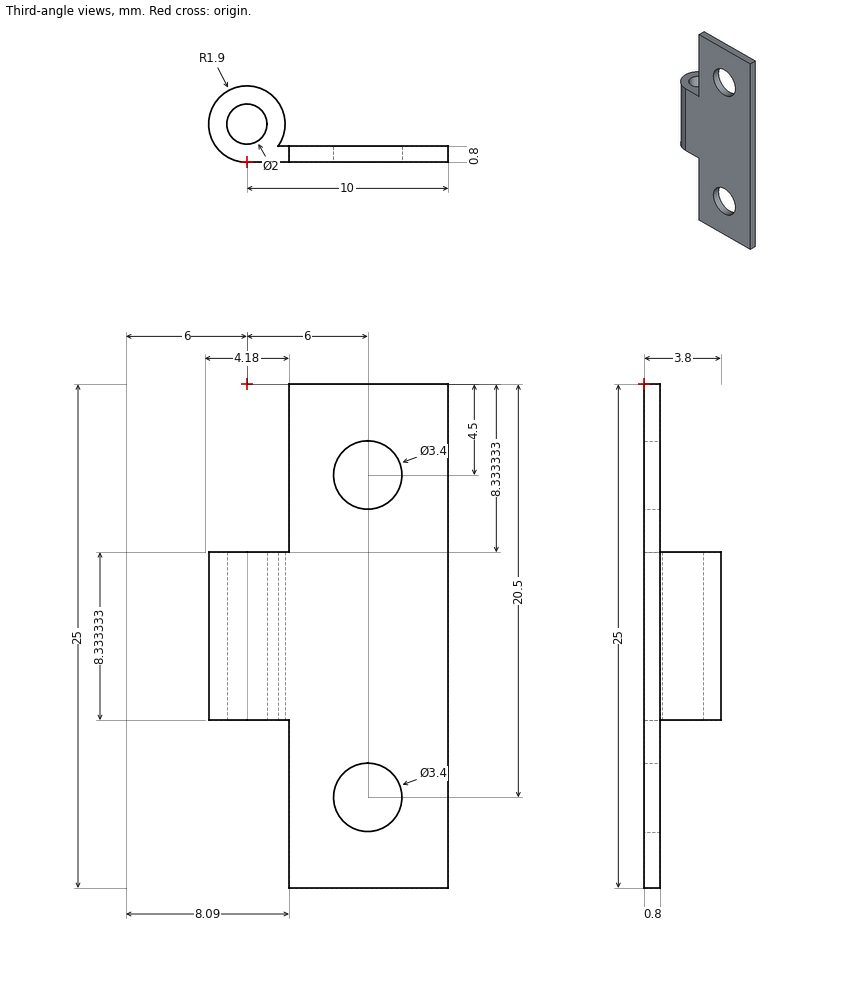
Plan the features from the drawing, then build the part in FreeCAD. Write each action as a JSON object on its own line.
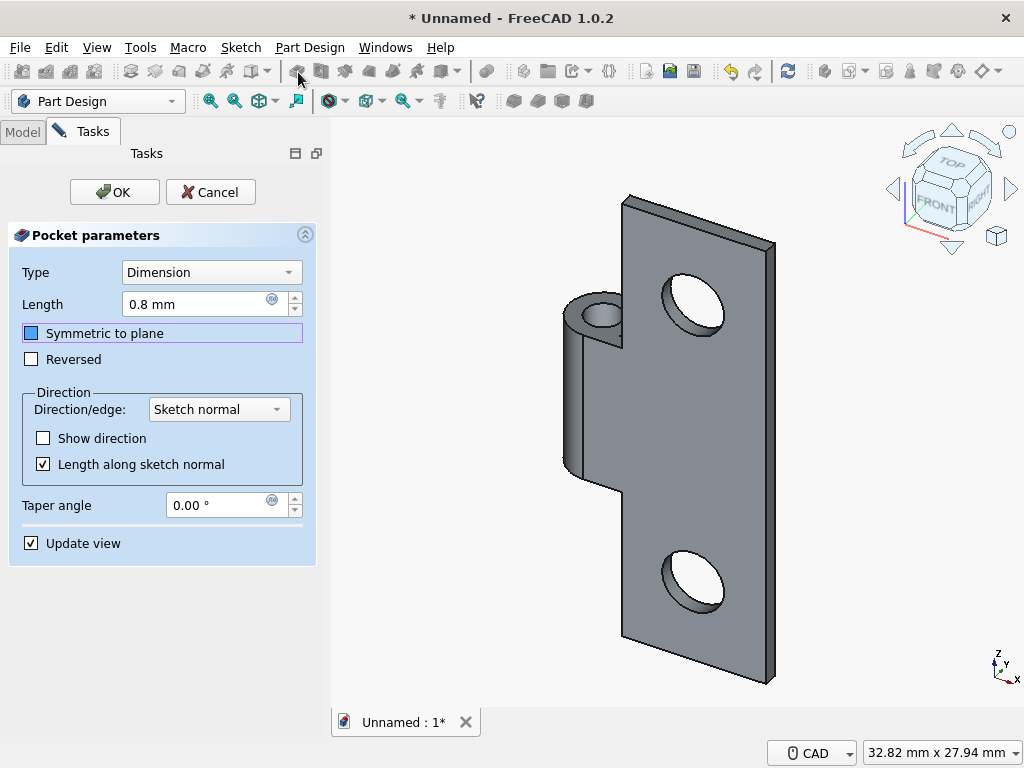
{"action": "left_click", "coordinate": [115, 192]}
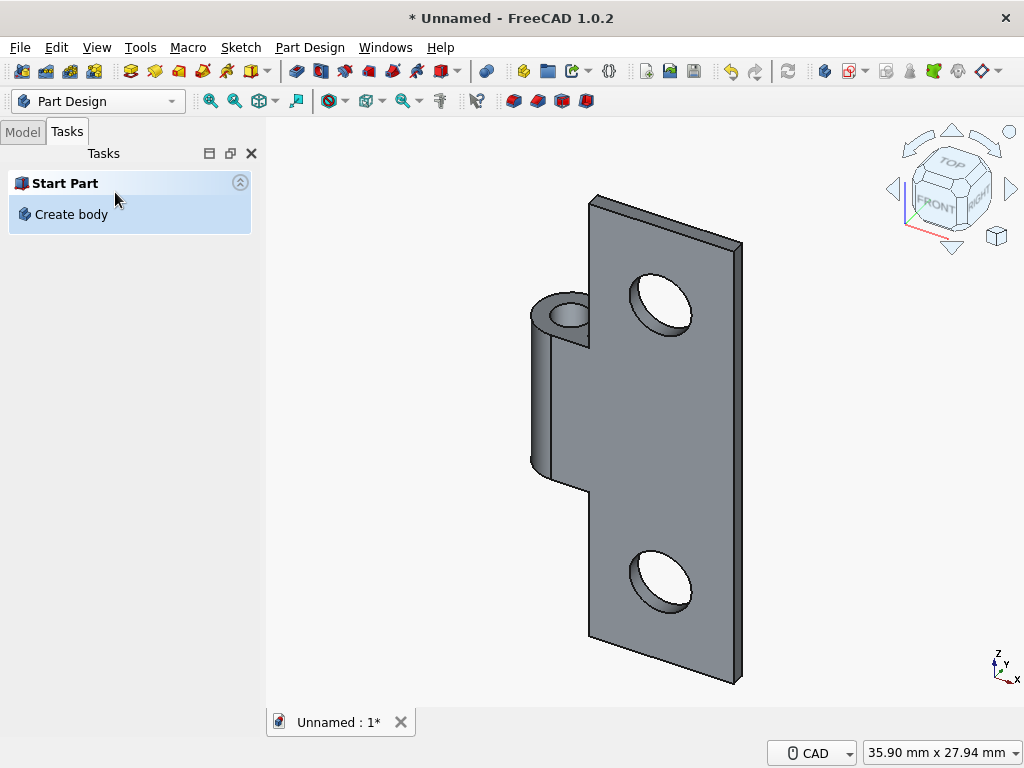
{"action": "key", "text": "0"}